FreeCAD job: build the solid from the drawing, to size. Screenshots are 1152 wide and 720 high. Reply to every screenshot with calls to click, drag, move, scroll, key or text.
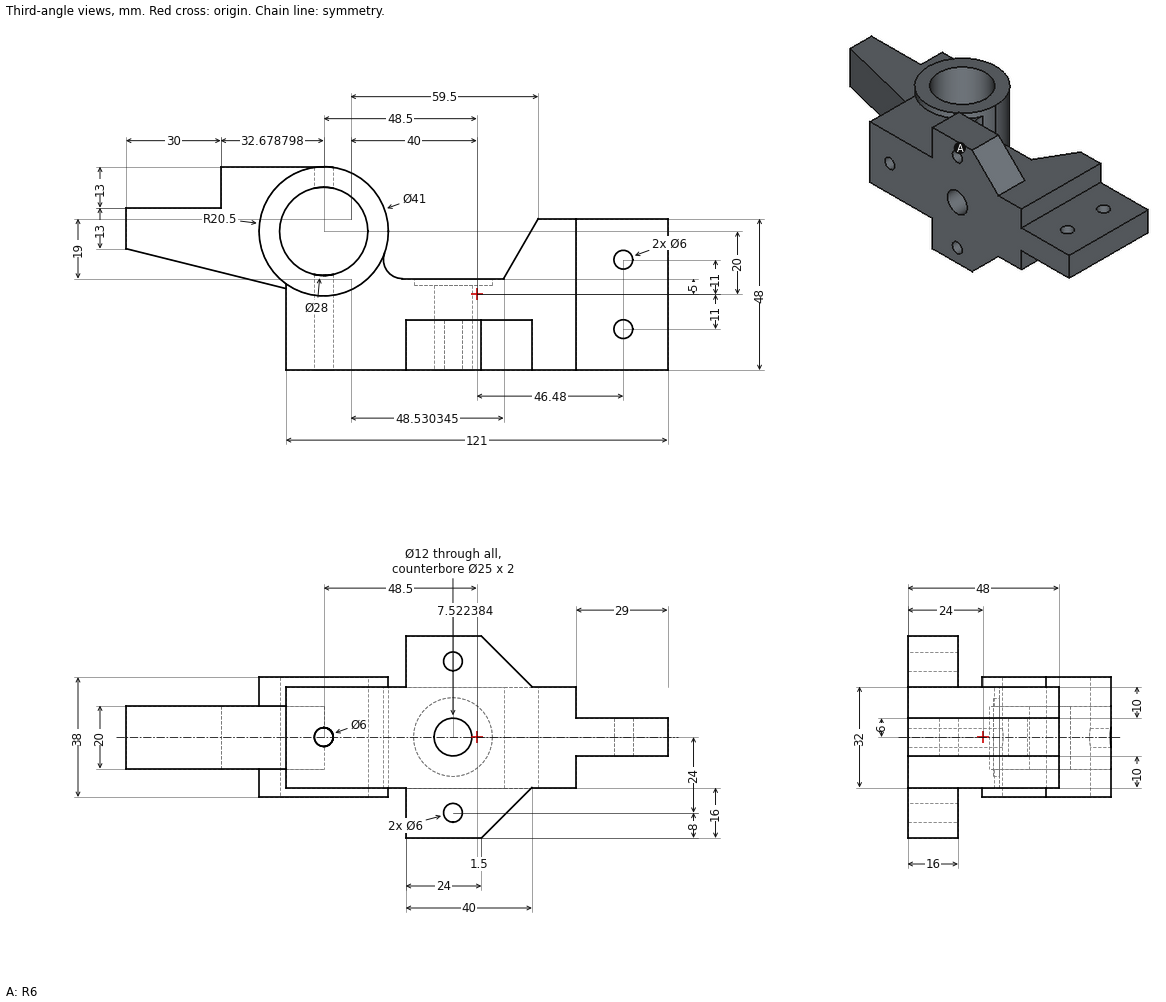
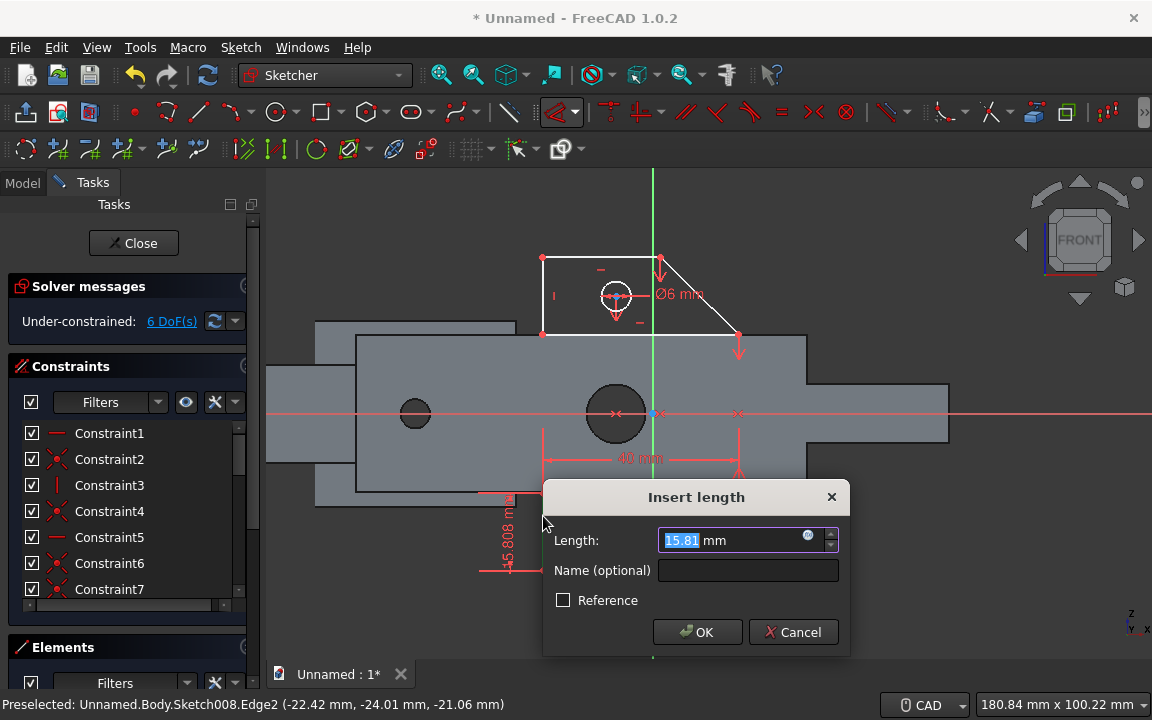
text(16)
key(Return)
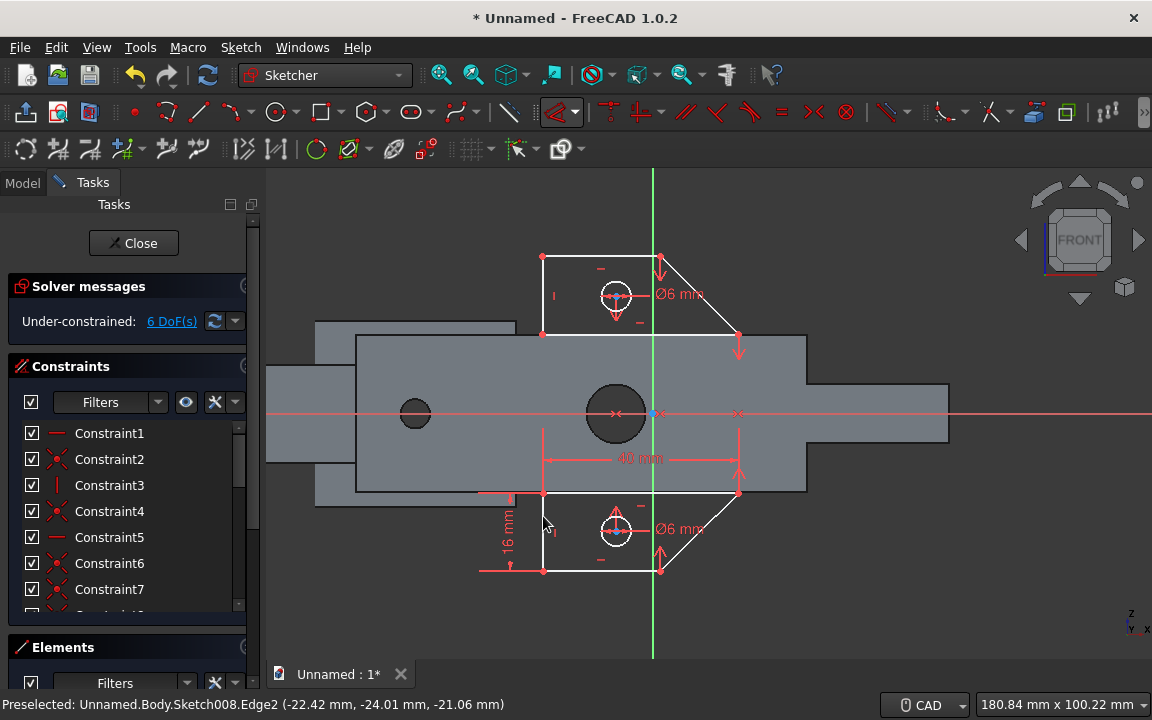
click(578, 571)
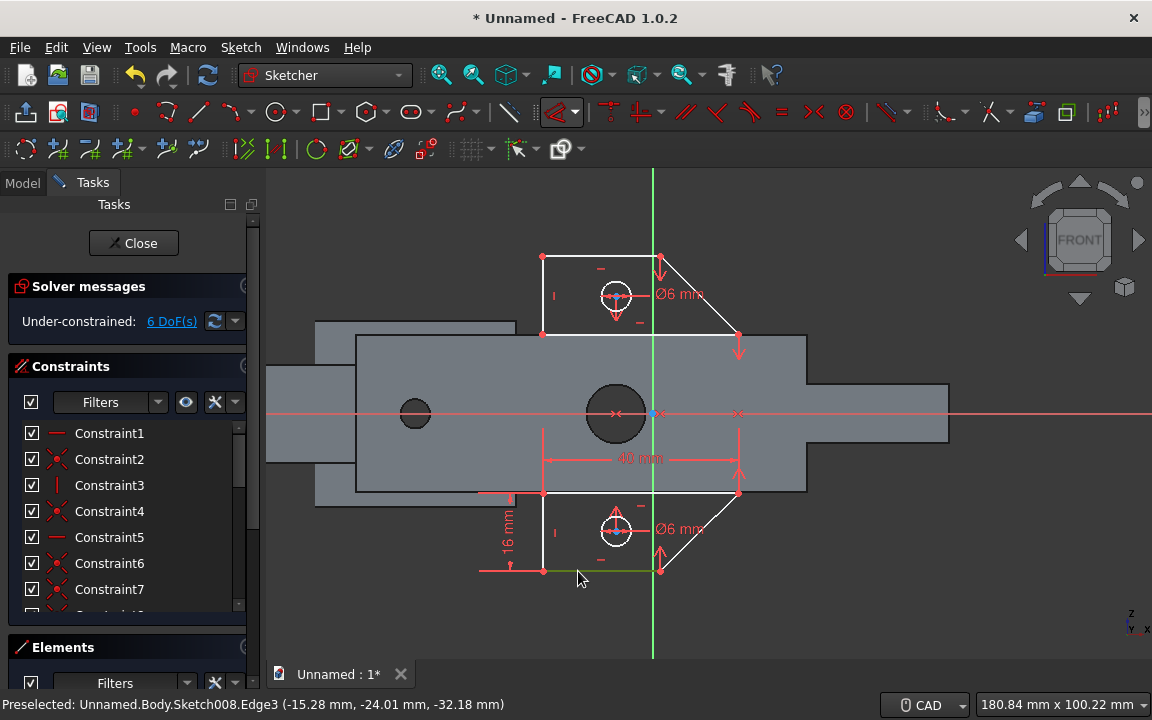
key(l)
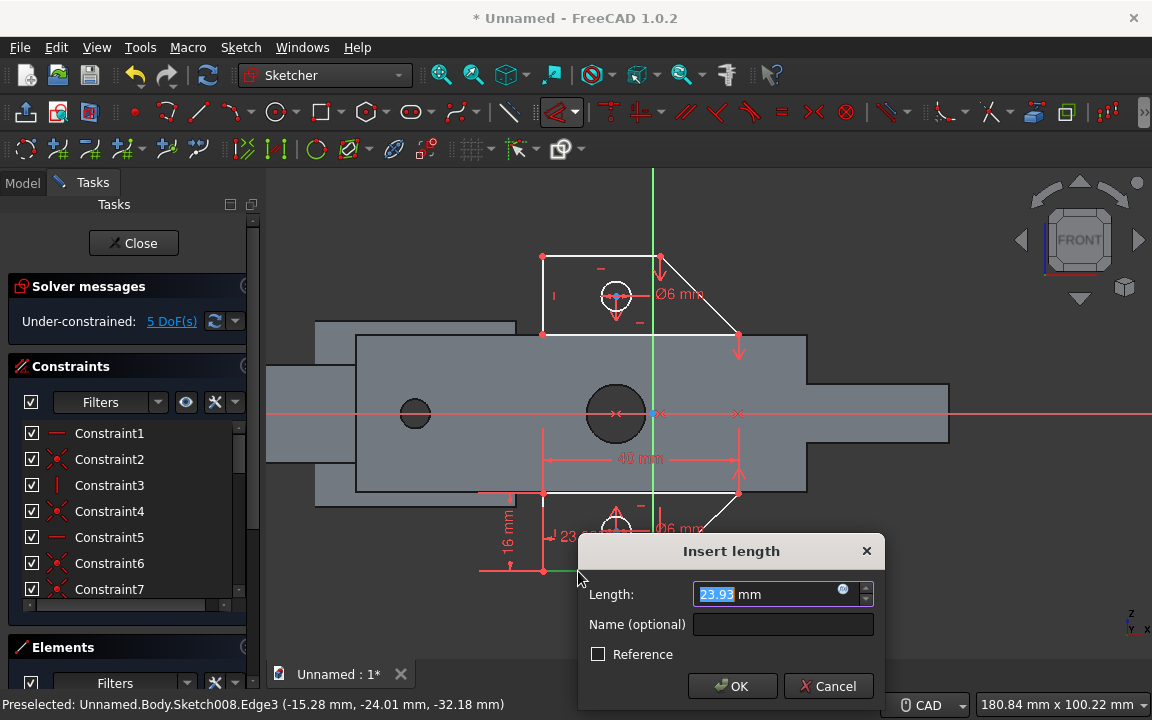
text(24)
key(Return)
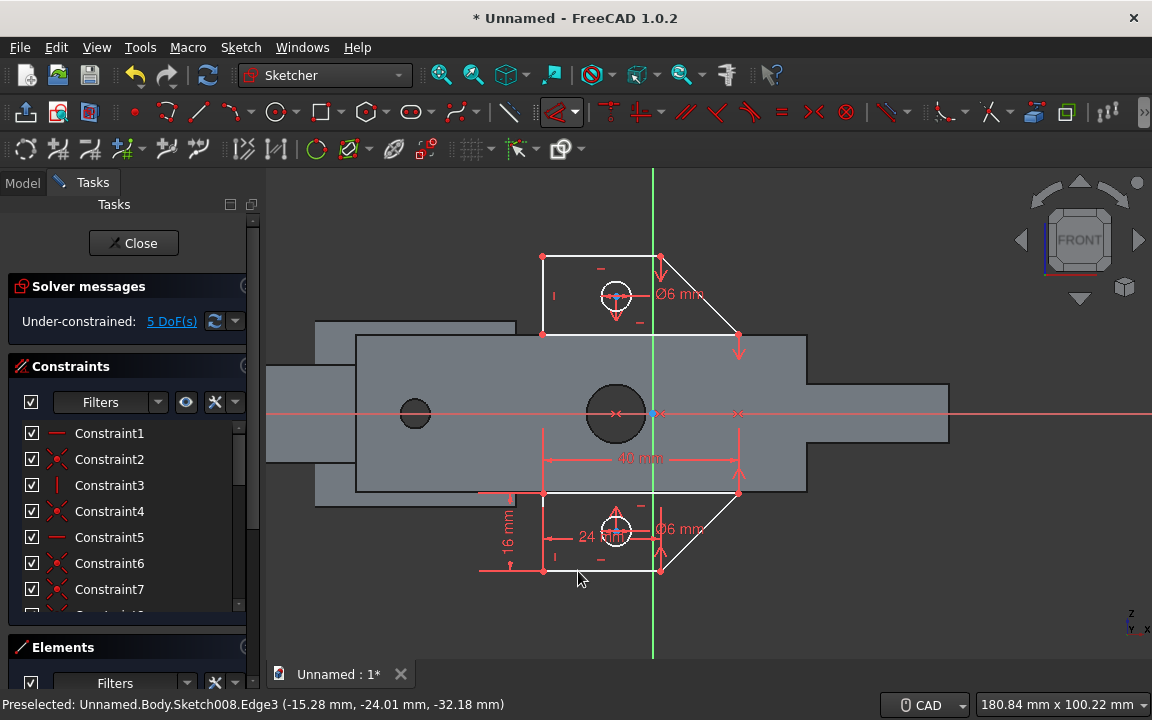
click(625, 256)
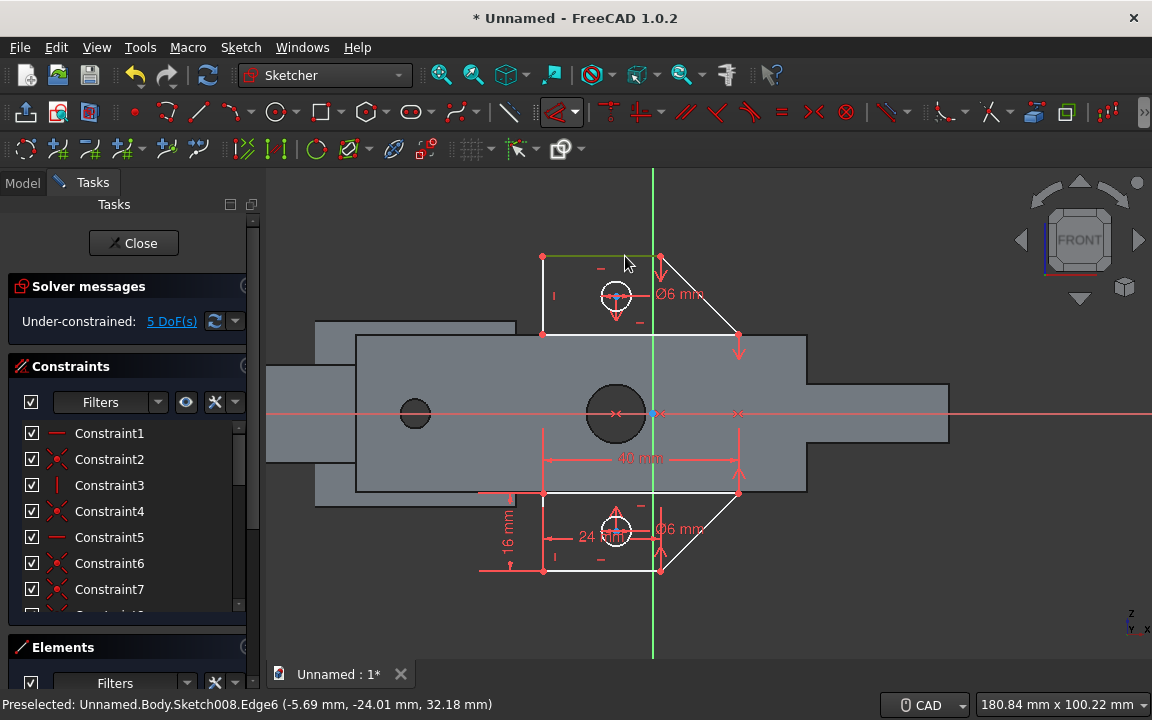
key(l)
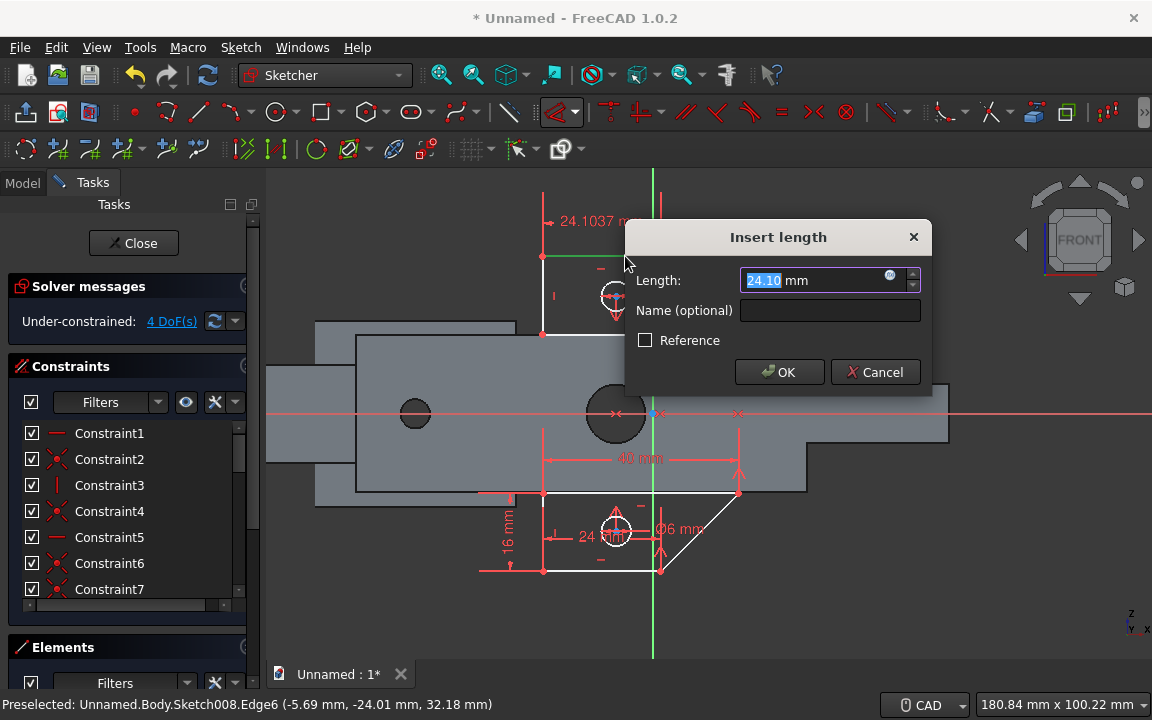
text(24)
key(Return)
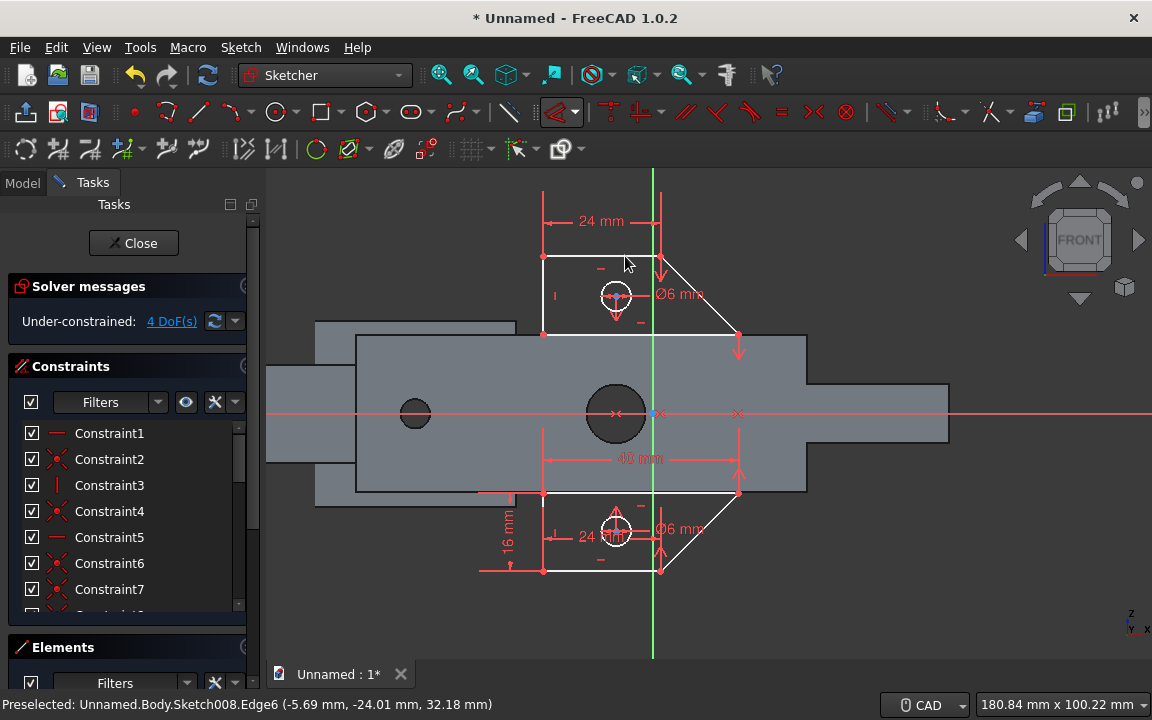
click(616, 531)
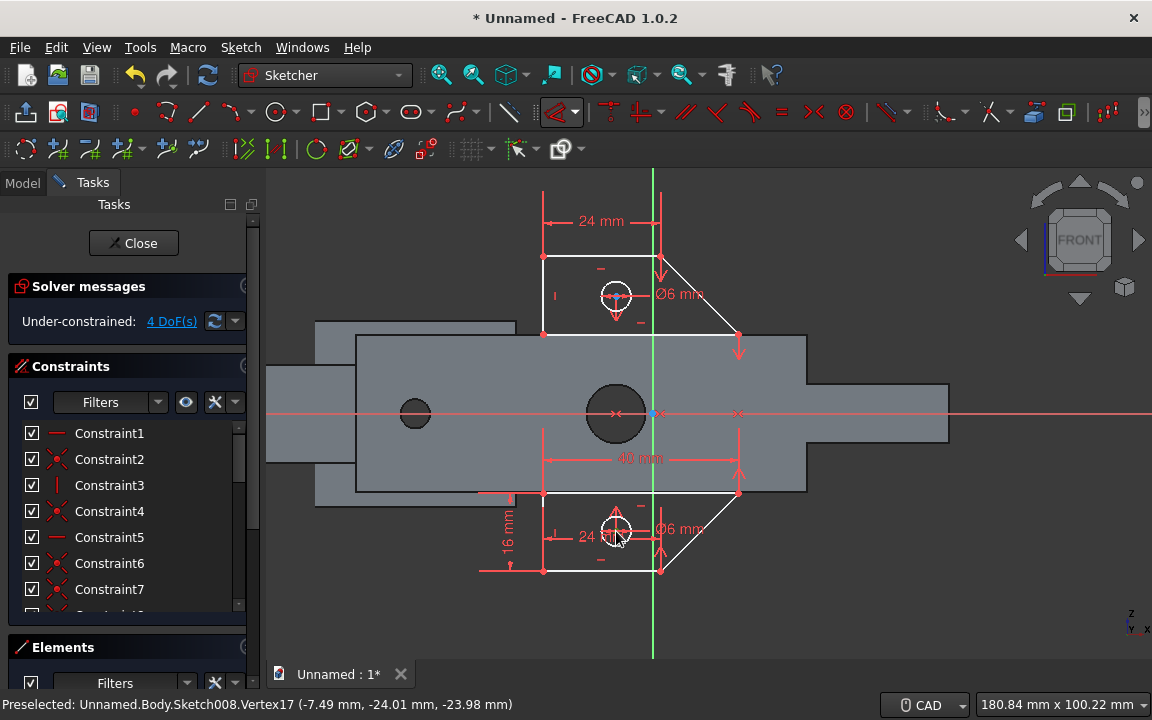
key(i)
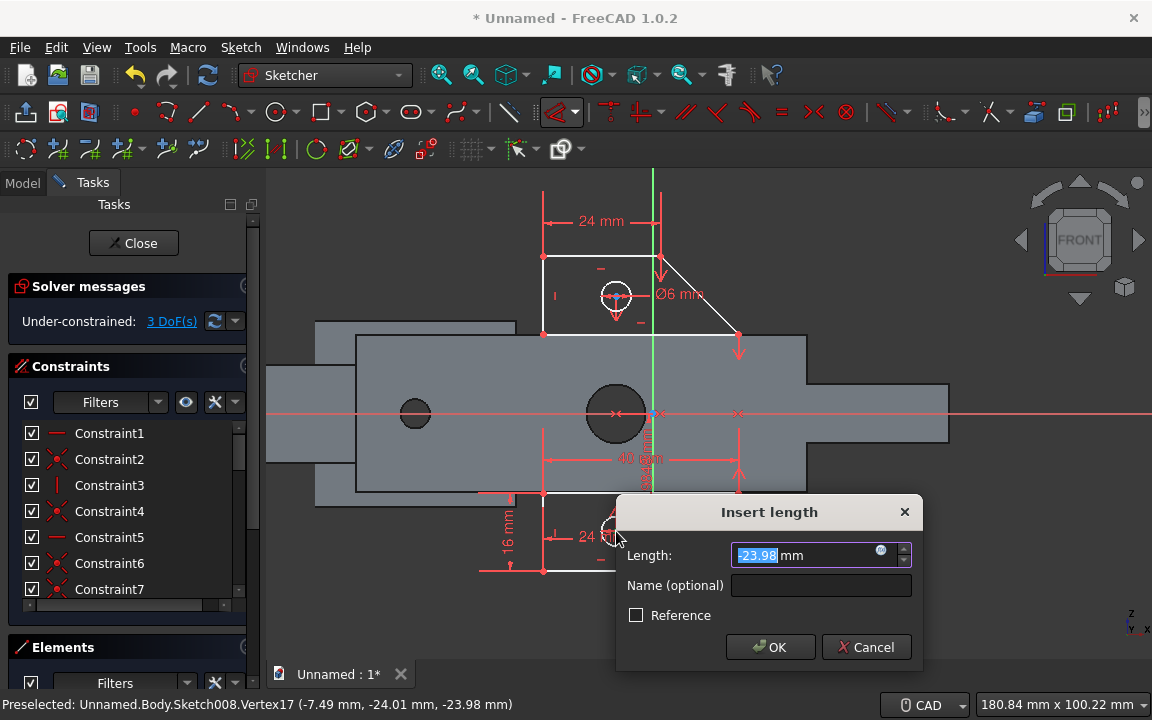
text(-24)
key(Return)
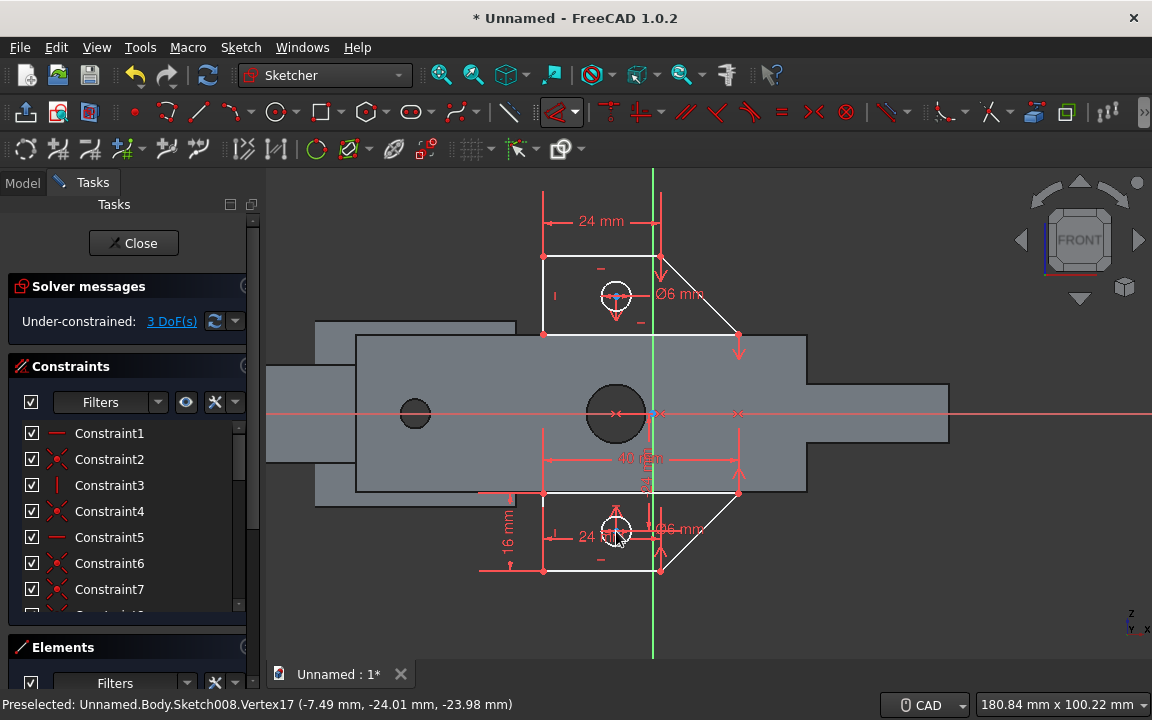
click(661, 571)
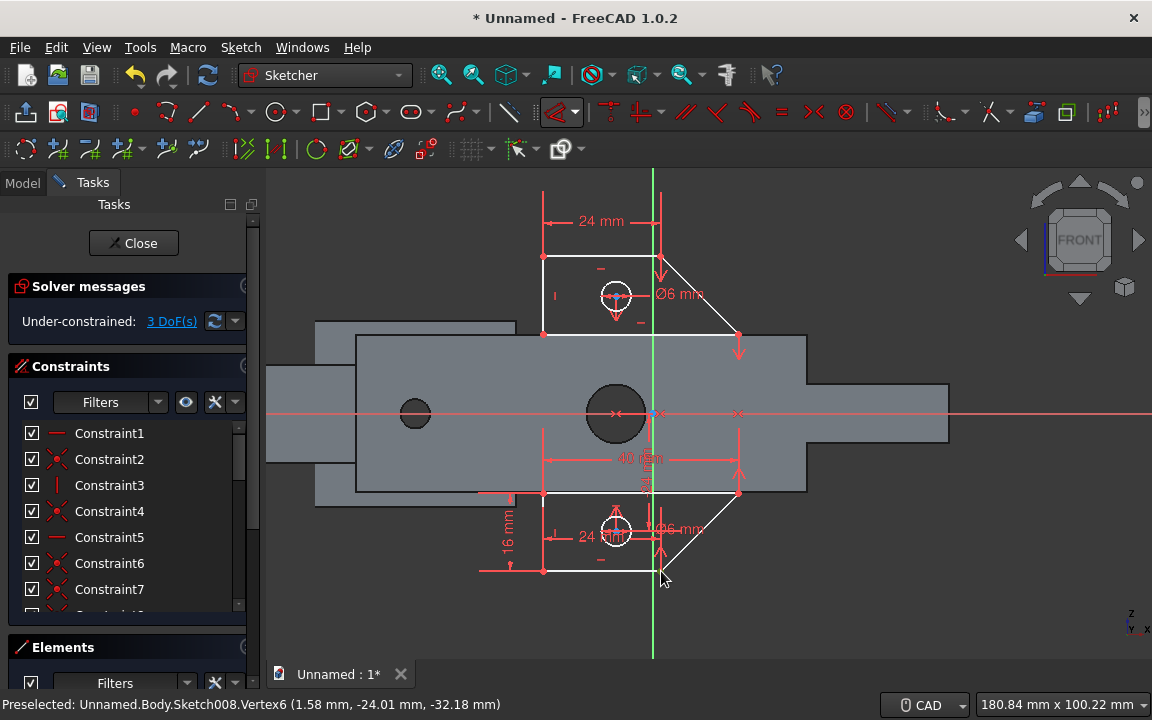
click(616, 531)